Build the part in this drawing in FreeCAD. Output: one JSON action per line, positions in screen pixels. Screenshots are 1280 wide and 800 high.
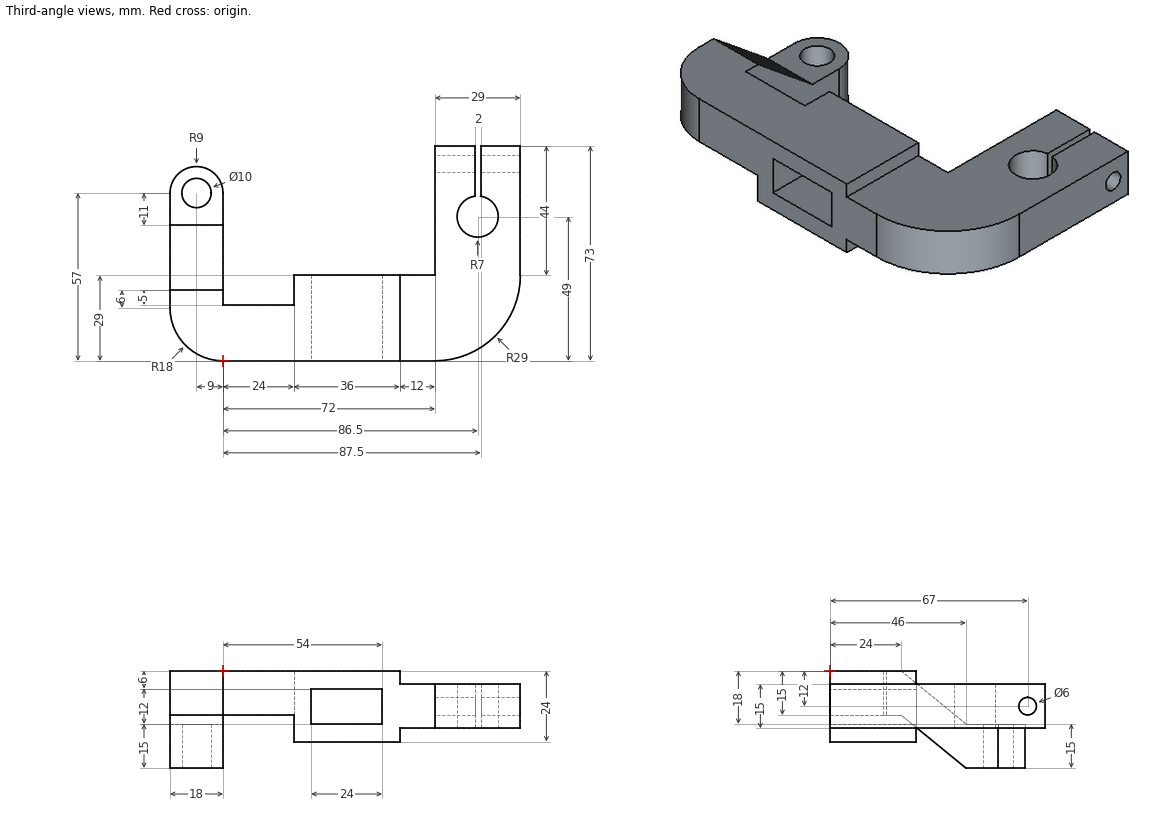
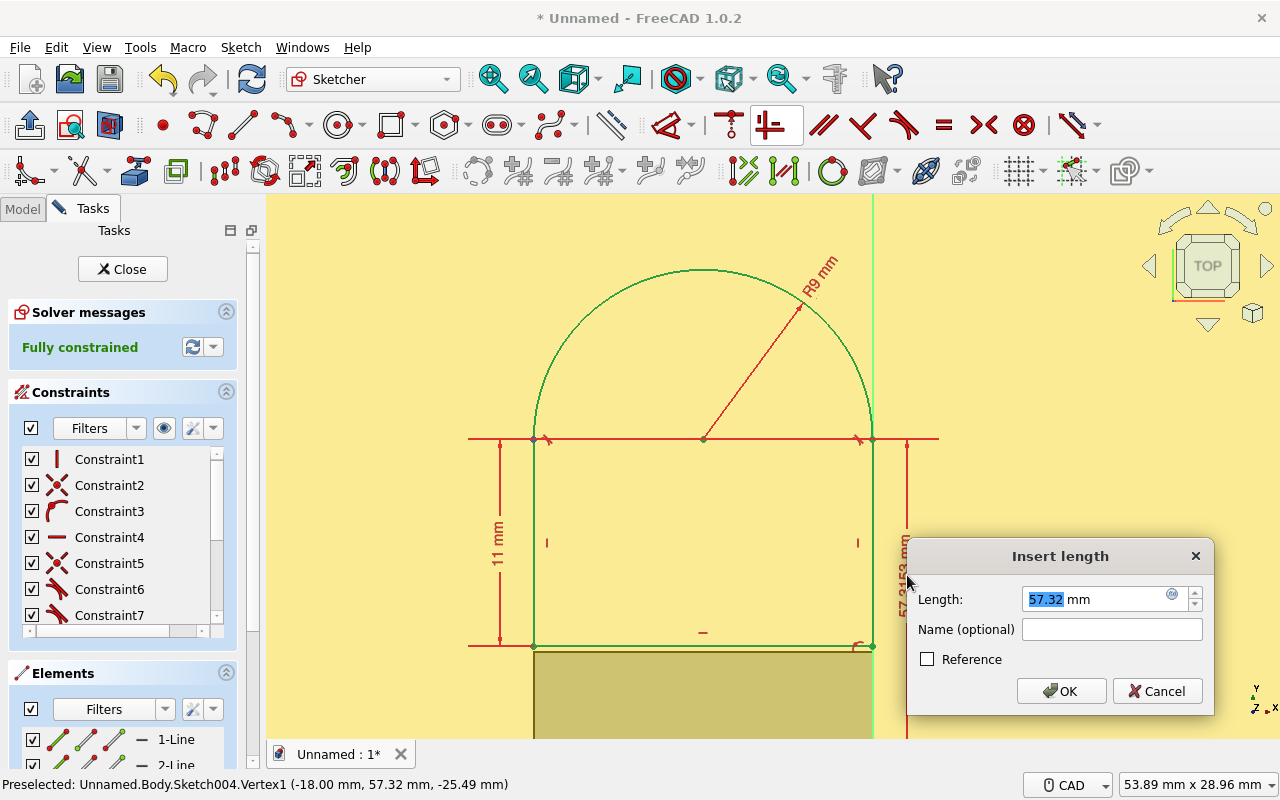
{"action": "type", "text": "57"}
{"action": "key", "text": "Return"}
{"action": "key", "text": "Escape"}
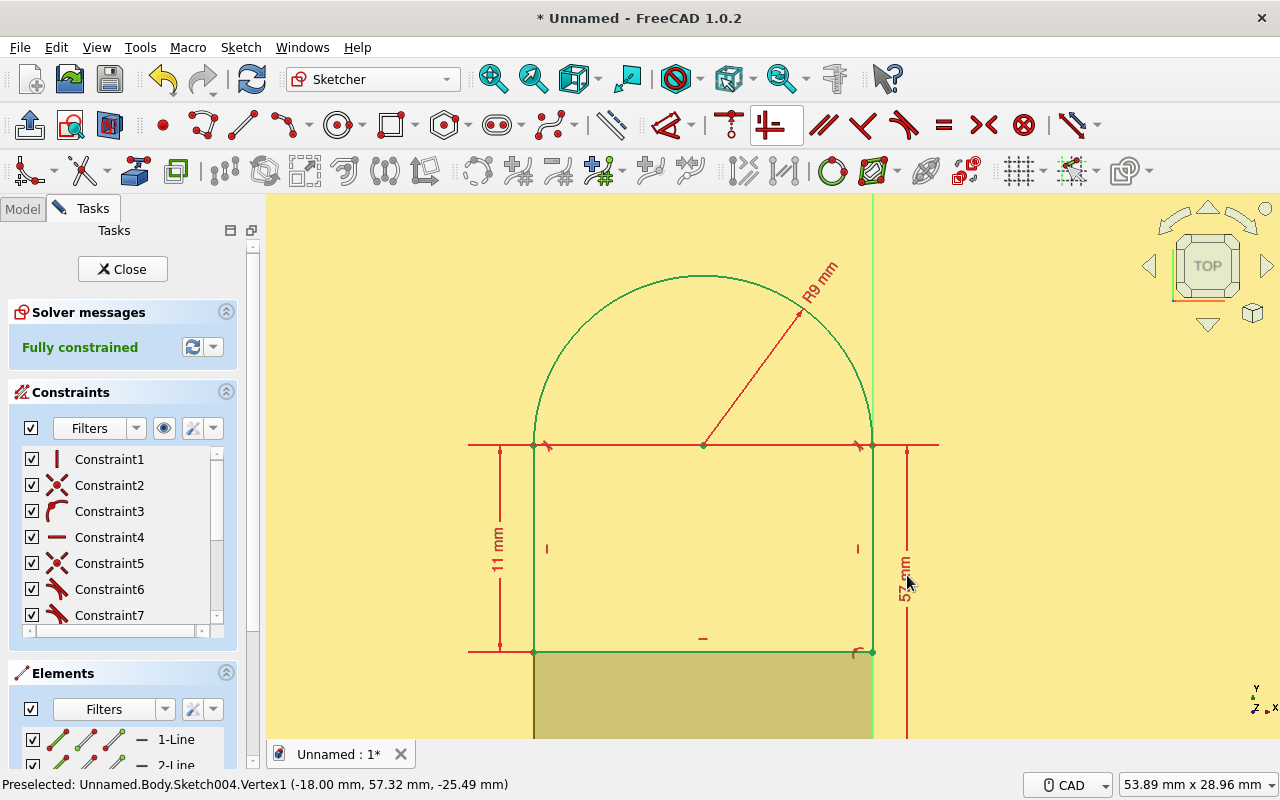
{"action": "left_click", "coordinate": [123, 269]}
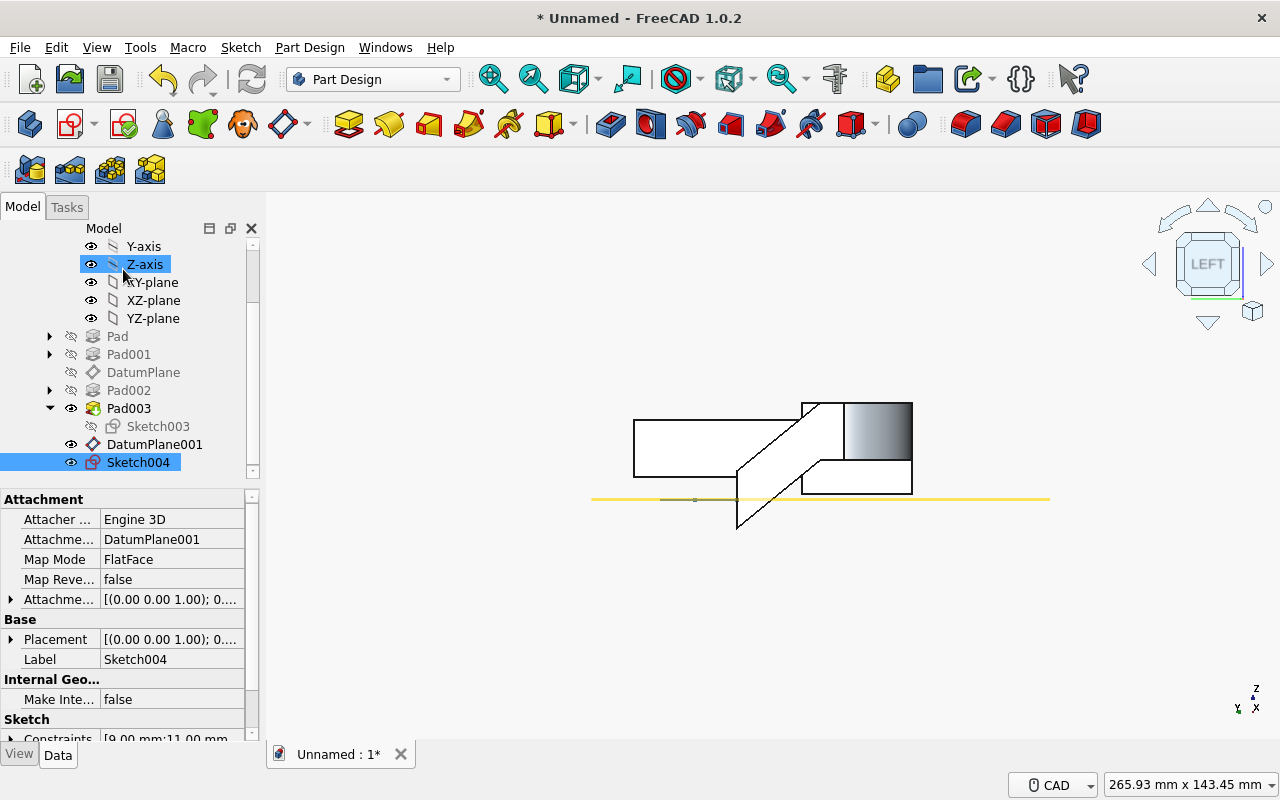
{"action": "left_click", "coordinate": [350, 124]}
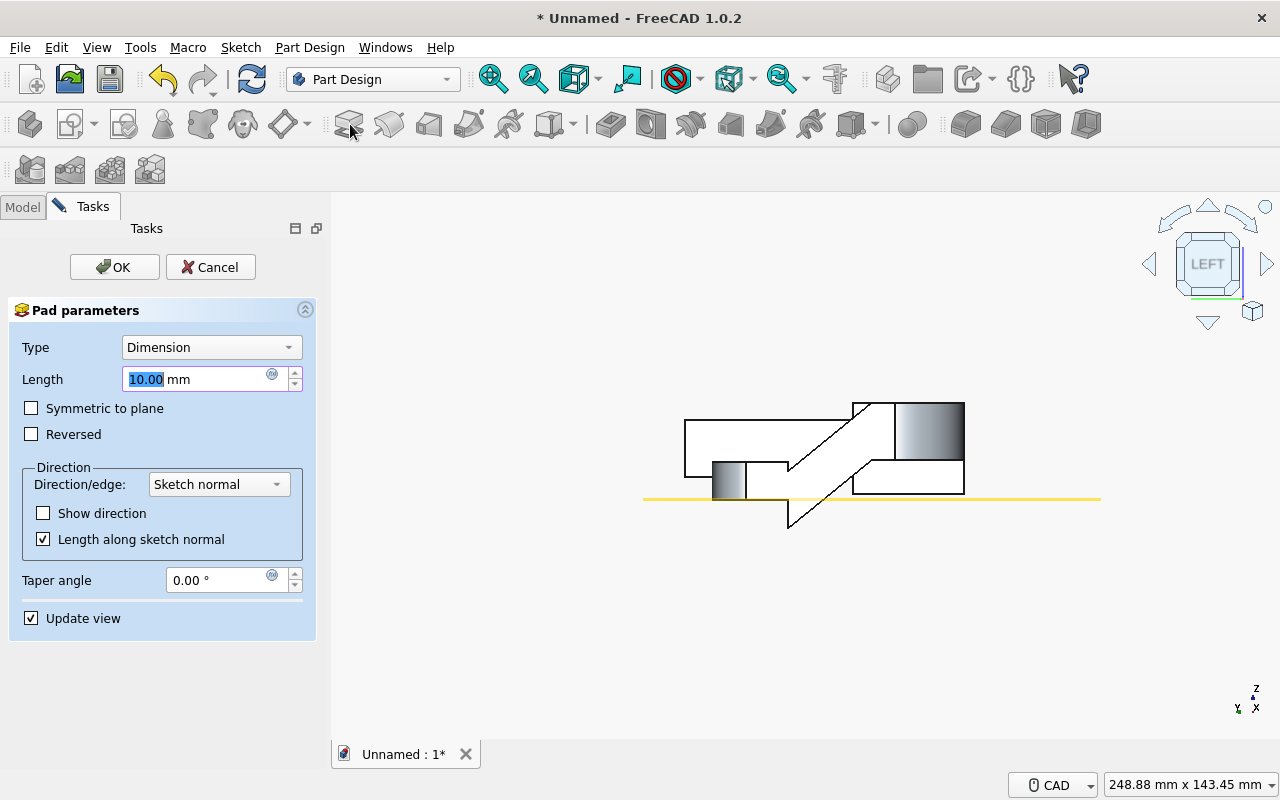
{"action": "type", "text": "15"}
{"action": "key", "text": "Tab"}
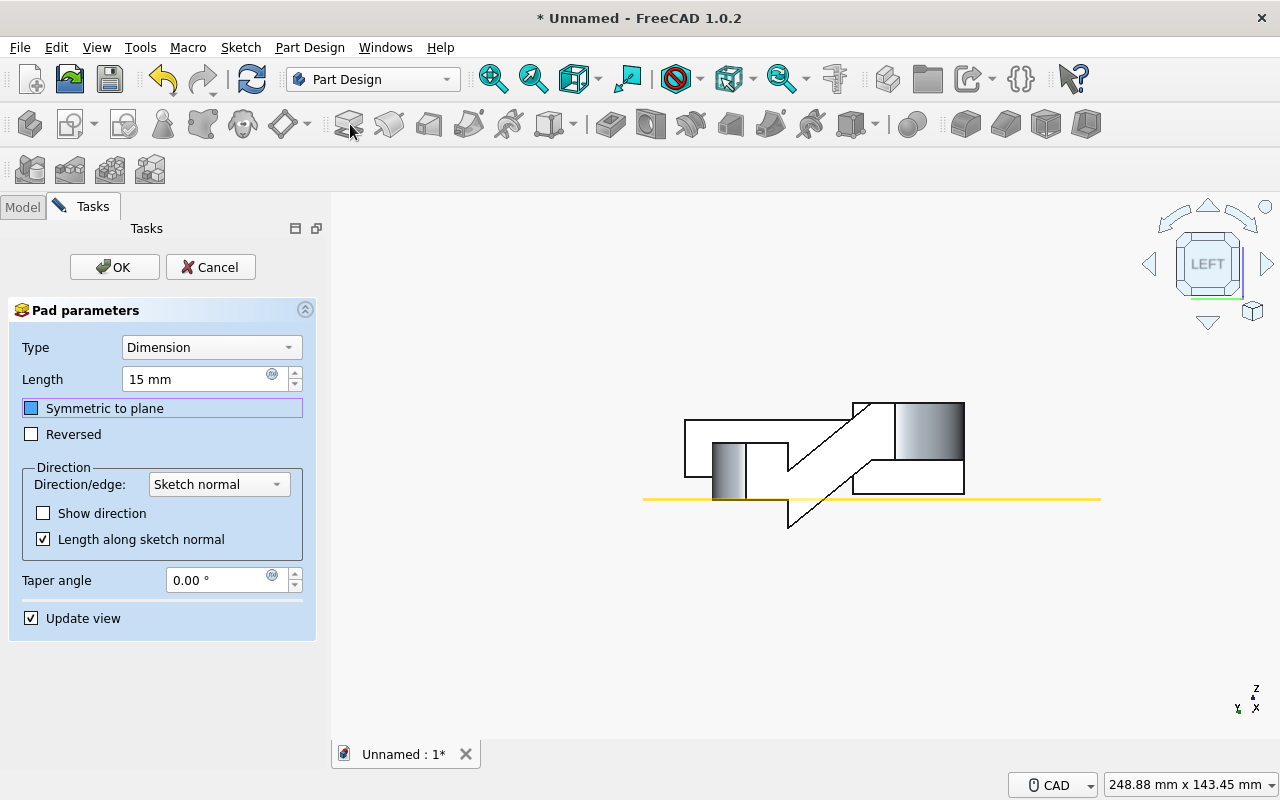
{"action": "left_click", "coordinate": [30, 408]}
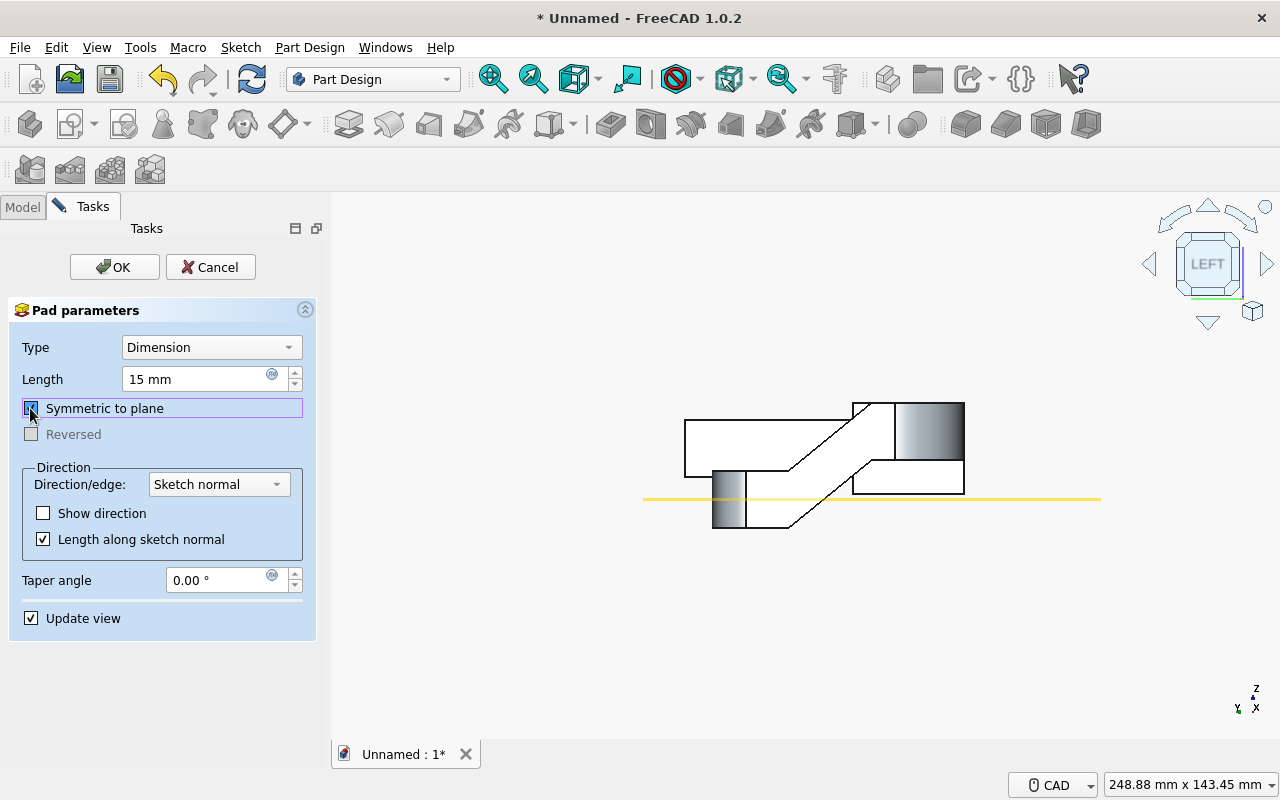
{"action": "left_click", "coordinate": [115, 267]}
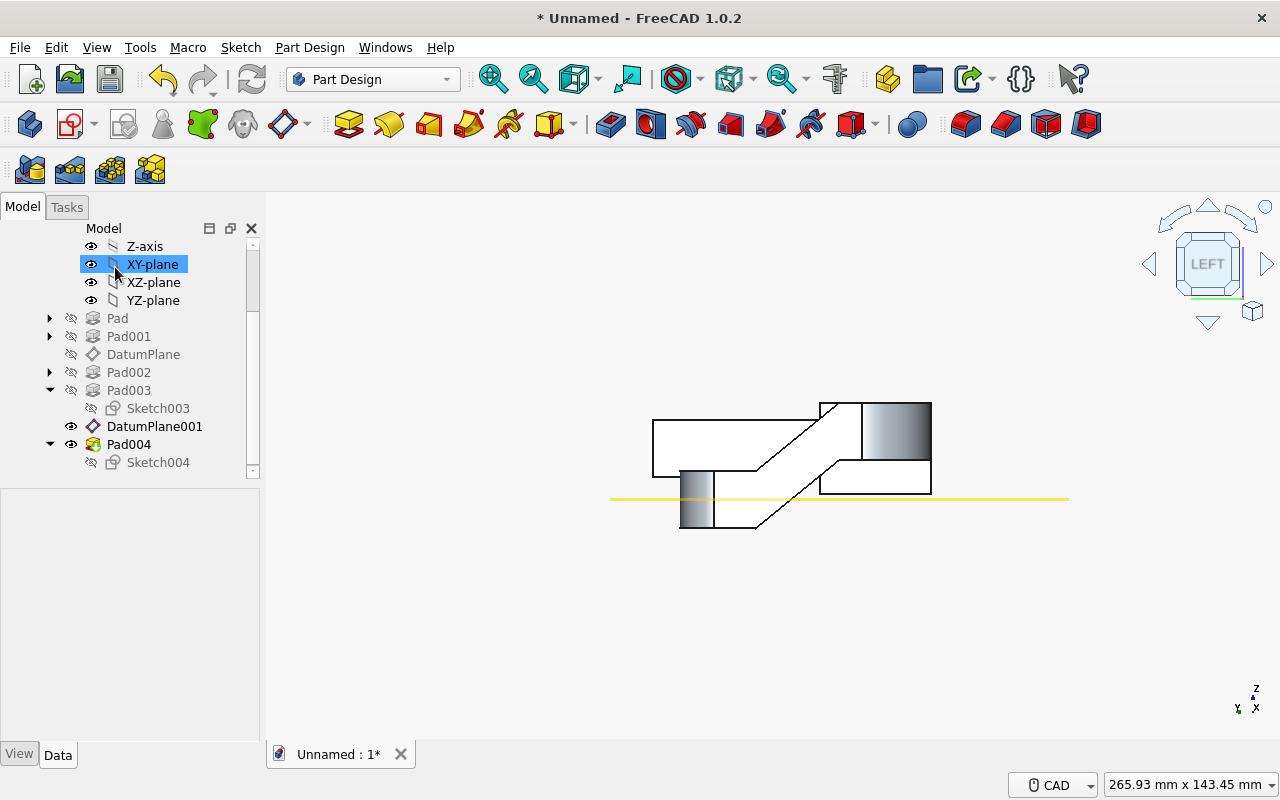
{"action": "left_click", "coordinate": [116, 426]}
{"action": "key", "text": "space"}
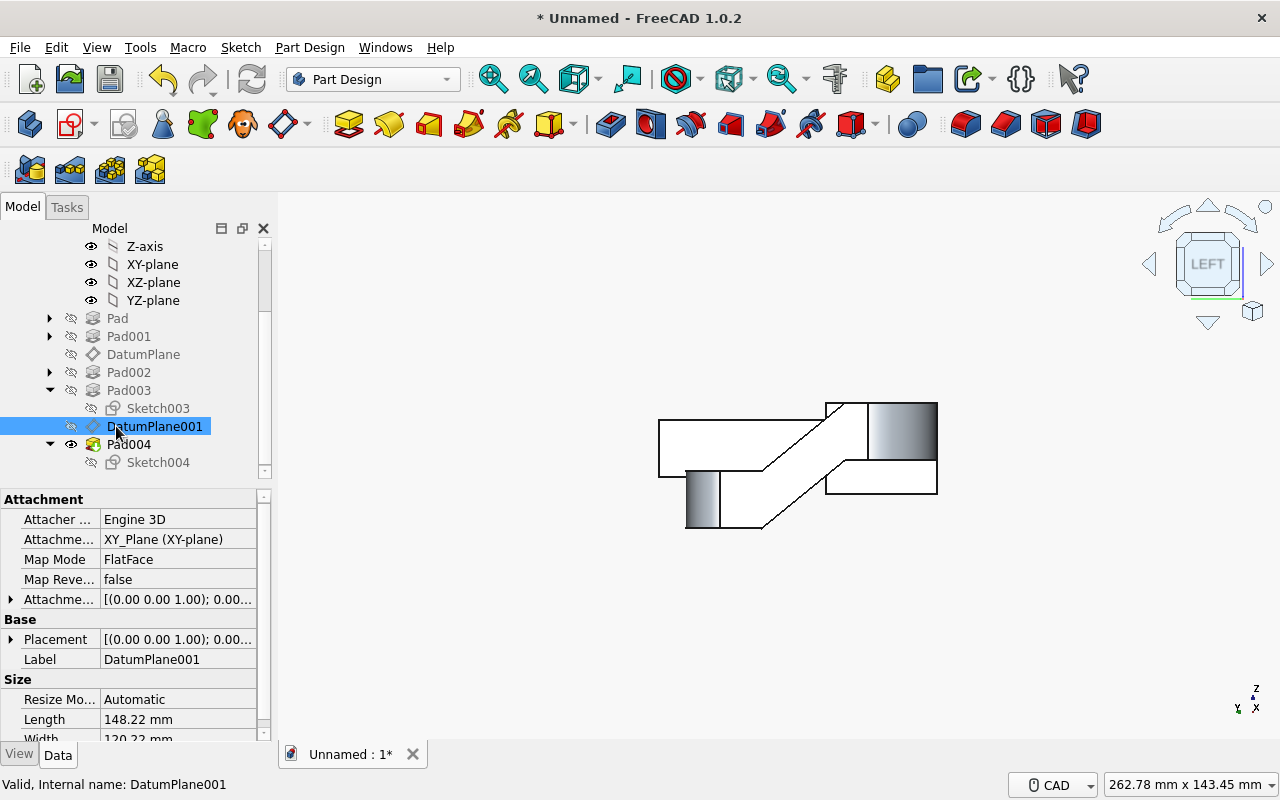
{"action": "left_click", "coordinate": [494, 80]}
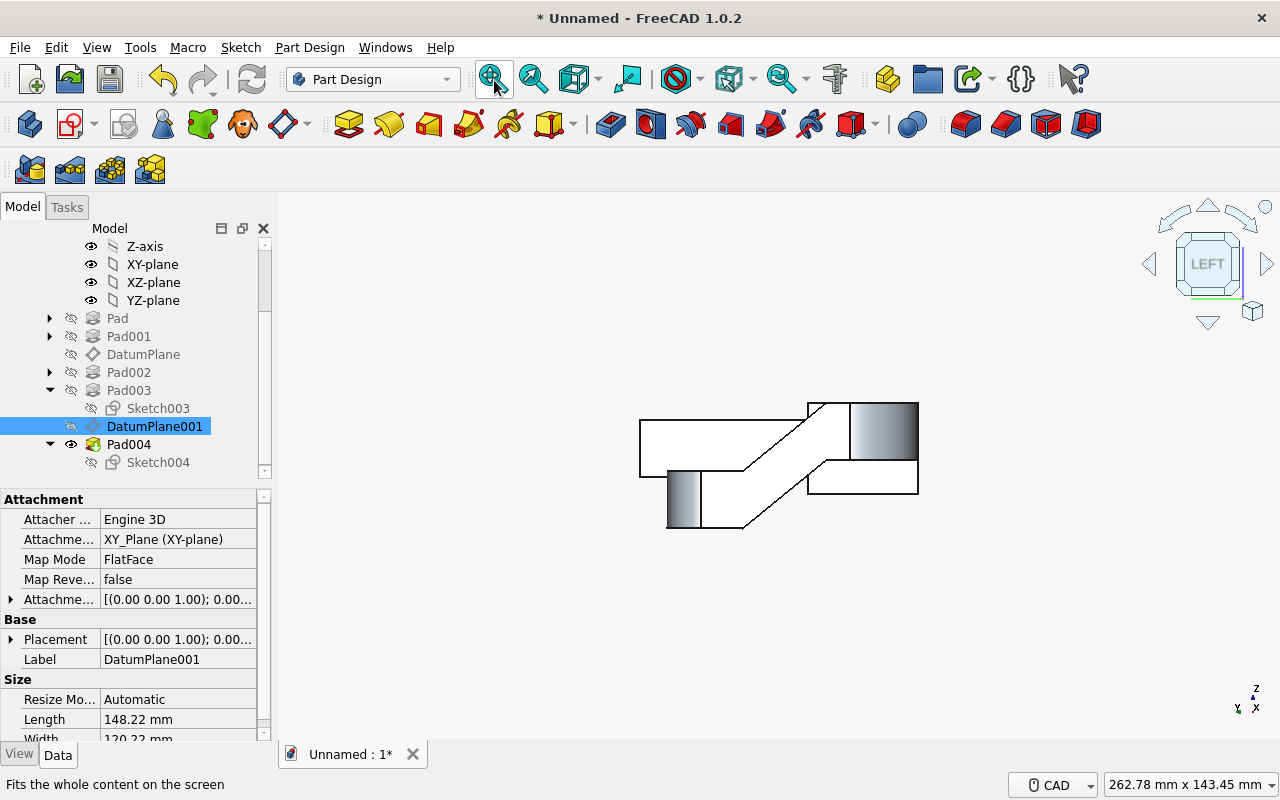
{"action": "key", "text": "0"}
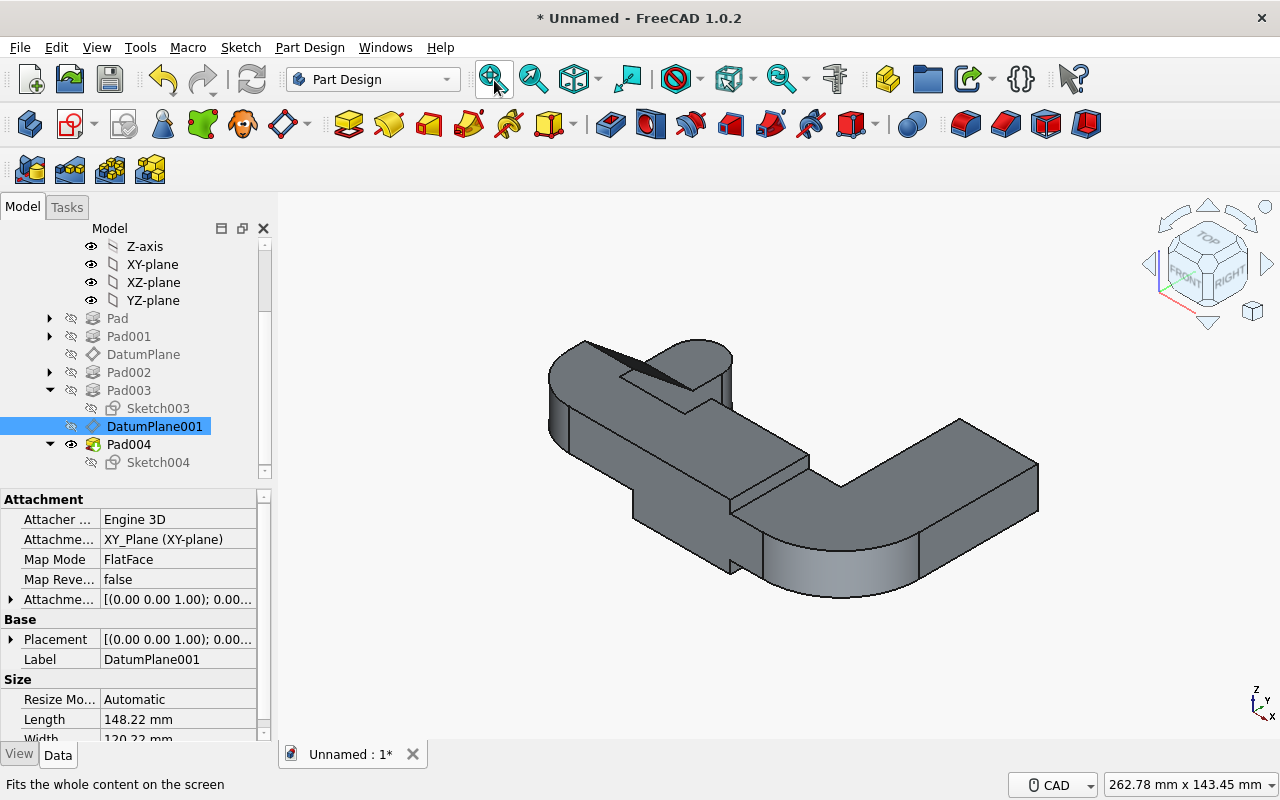
{"action": "left_click", "coordinate": [695, 360]}